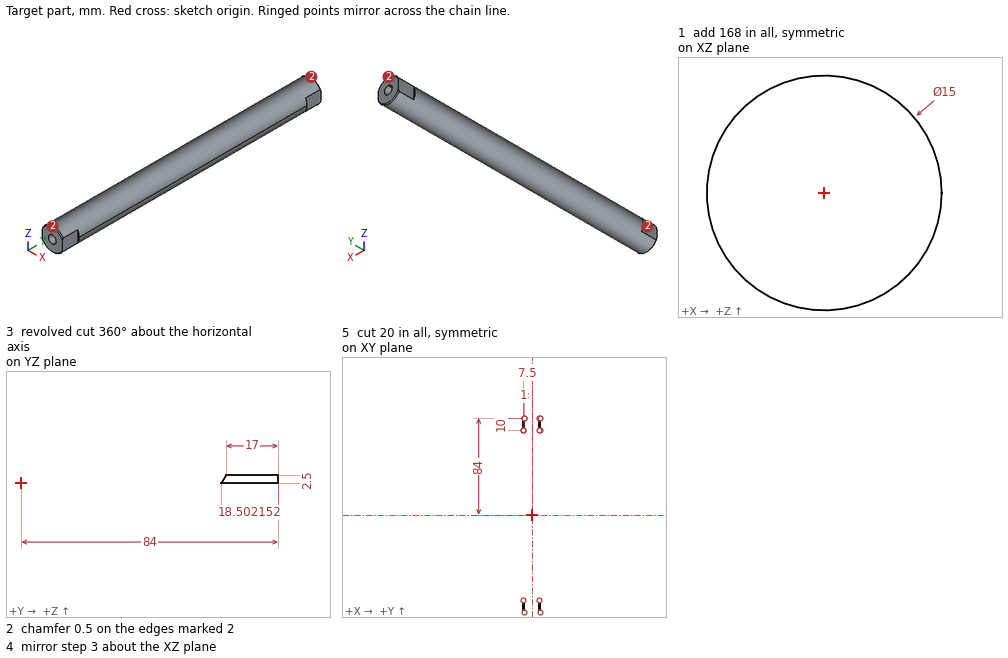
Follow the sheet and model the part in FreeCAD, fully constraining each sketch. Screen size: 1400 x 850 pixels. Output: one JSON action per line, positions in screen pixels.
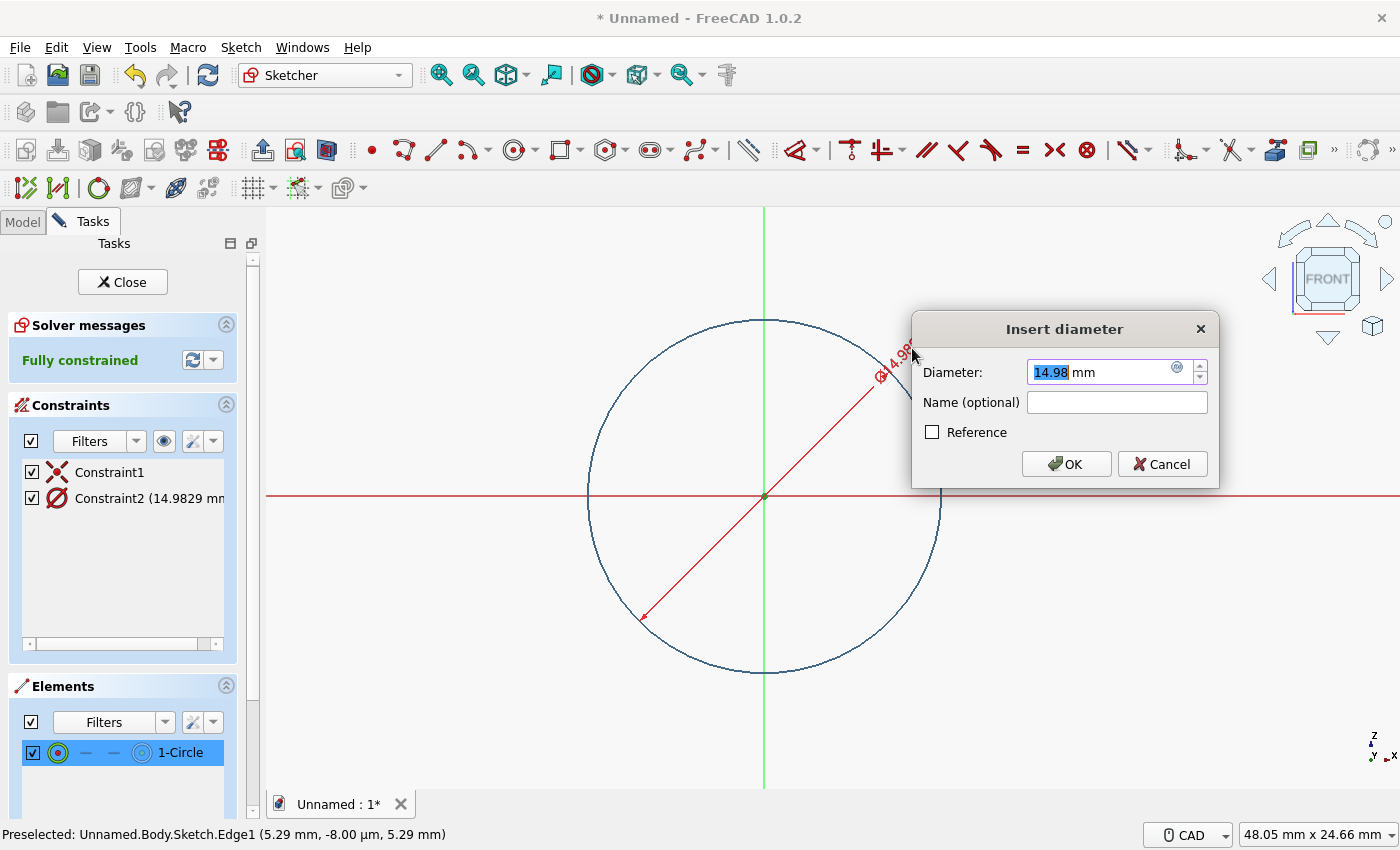
{"action": "type", "text": "15"}
{"action": "key", "text": "Return"}
{"action": "key", "text": "Escape"}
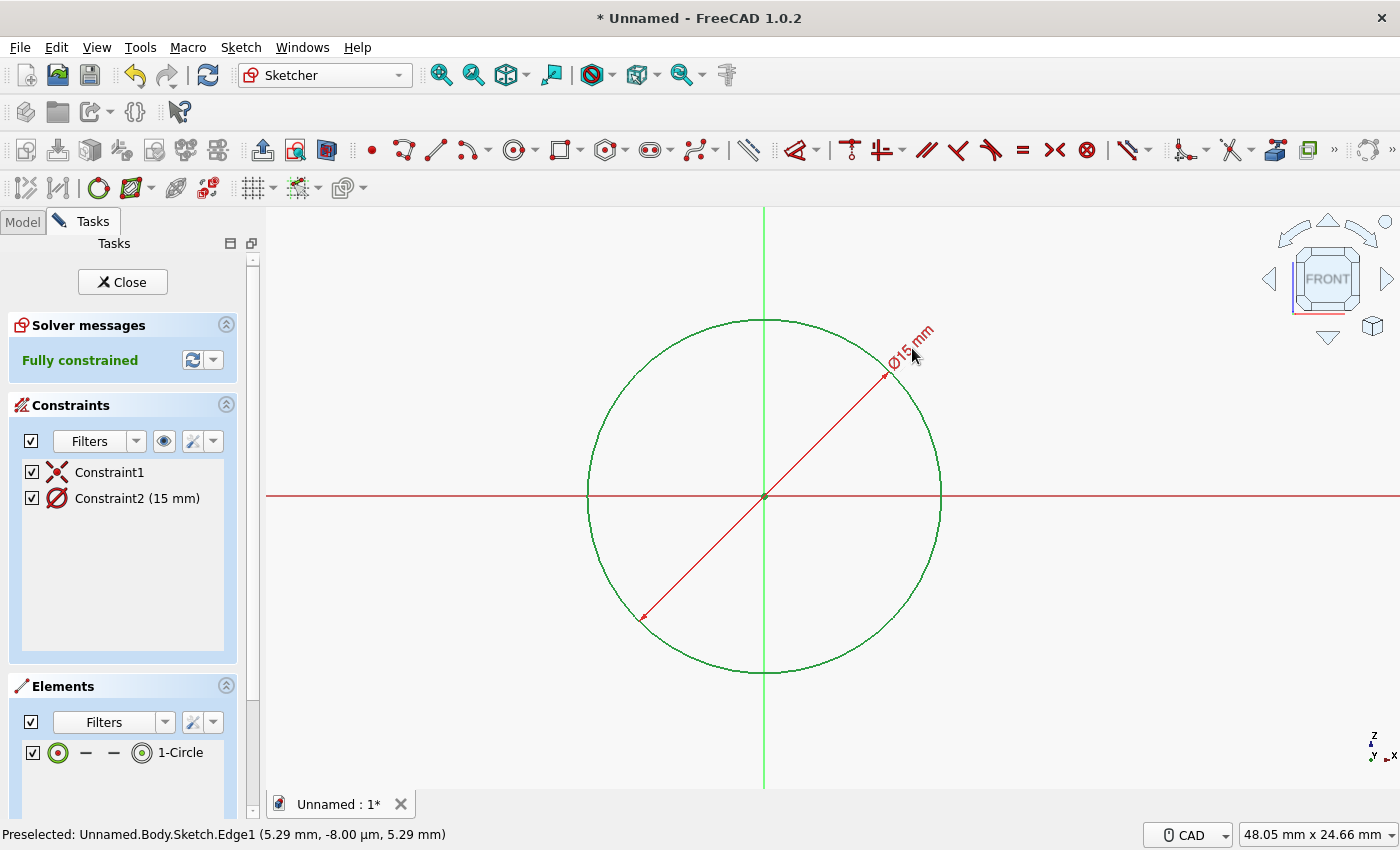
{"action": "left_click", "coordinate": [123, 282]}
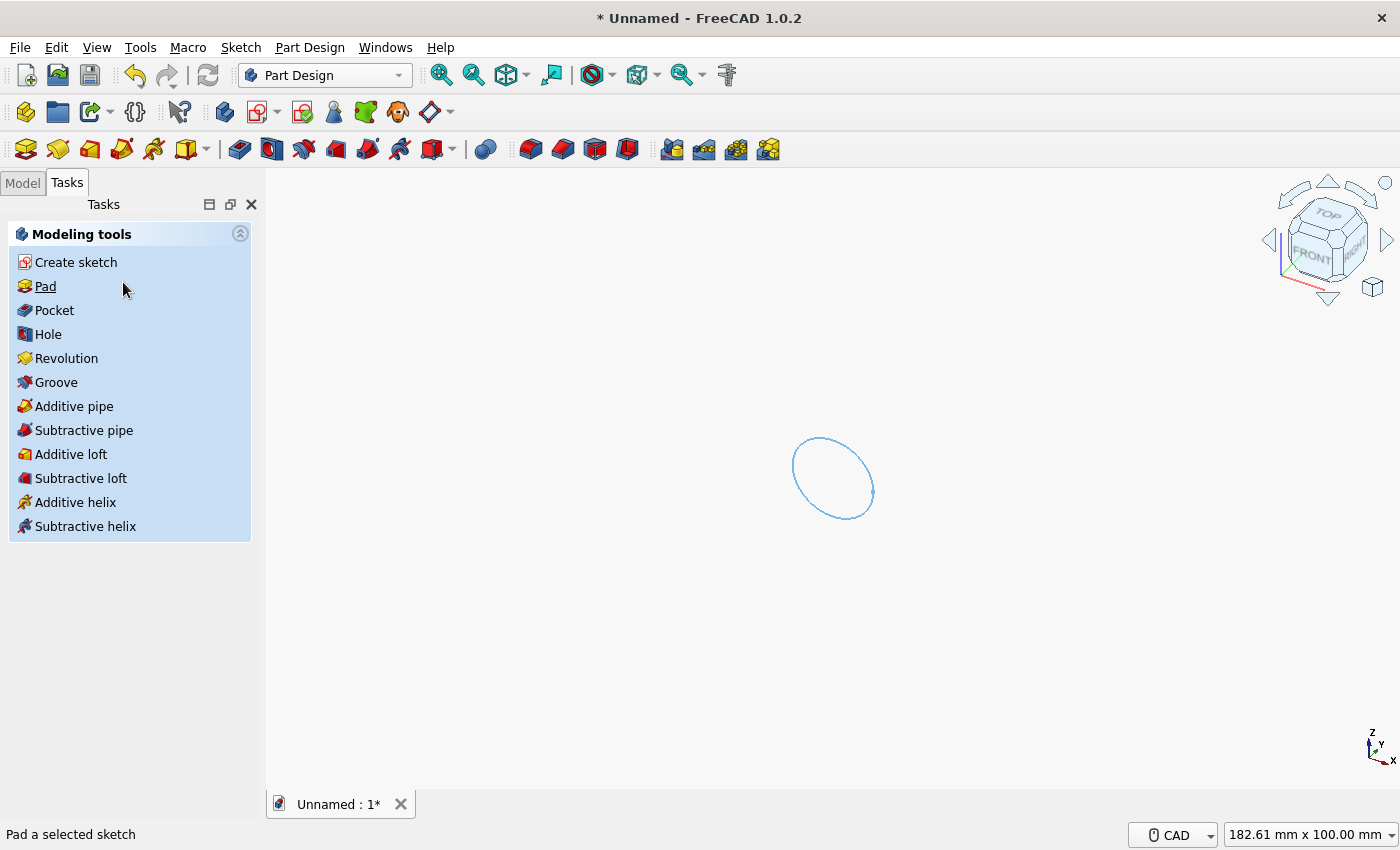
{"action": "left_click", "coordinate": [26, 150]}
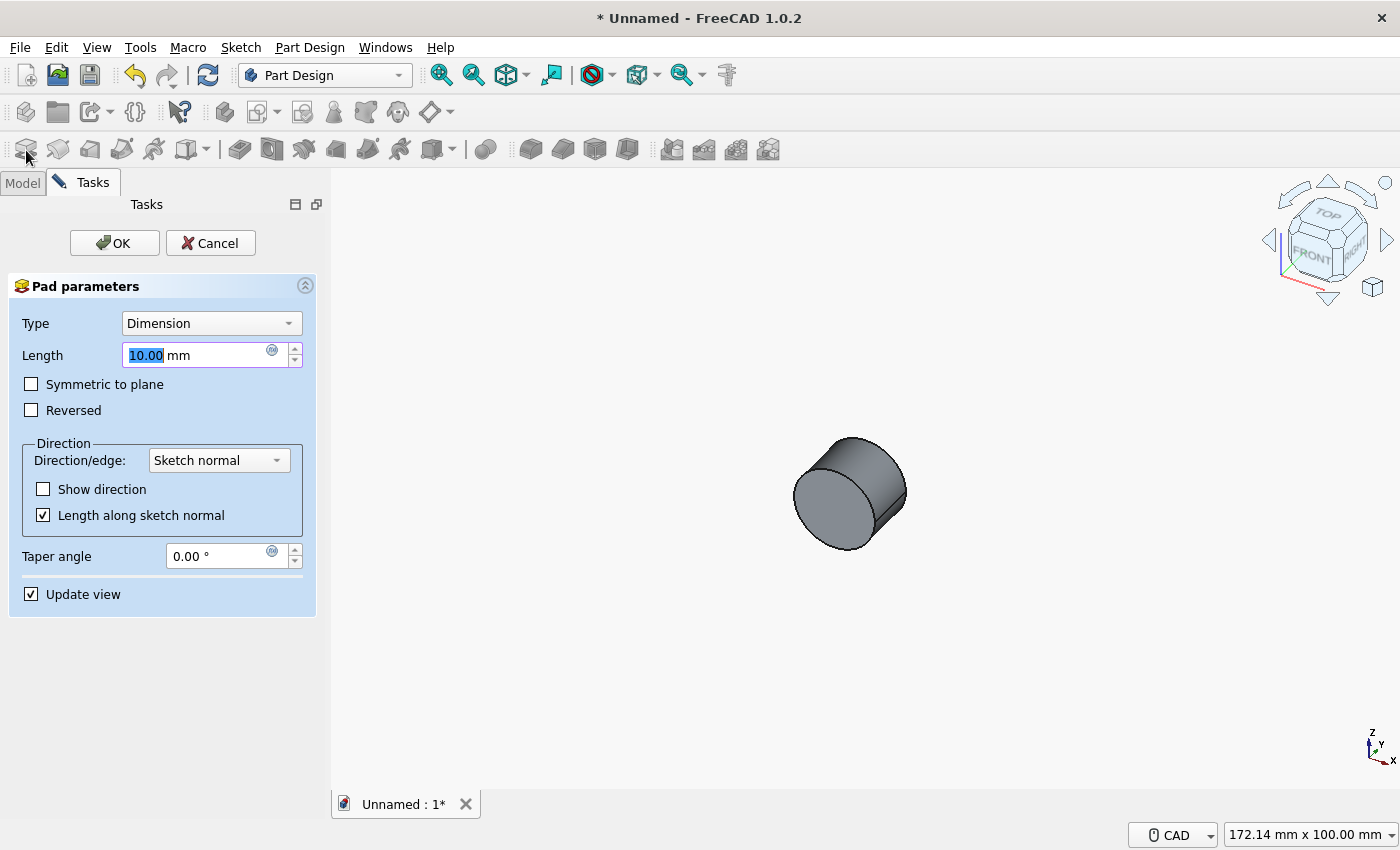
{"action": "type", "text": "168"}
{"action": "key", "text": "Tab"}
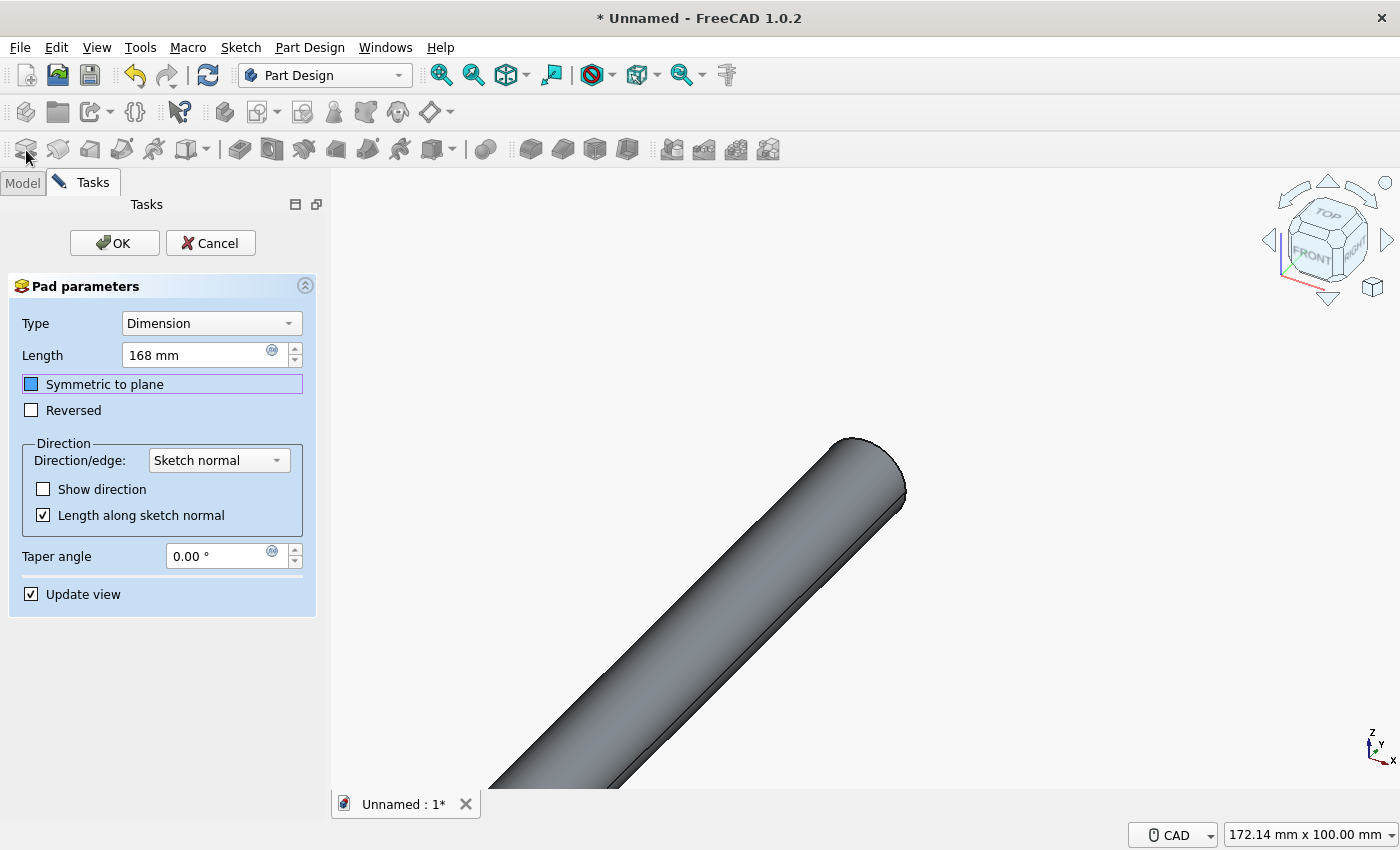
{"action": "left_click", "coordinate": [30, 384]}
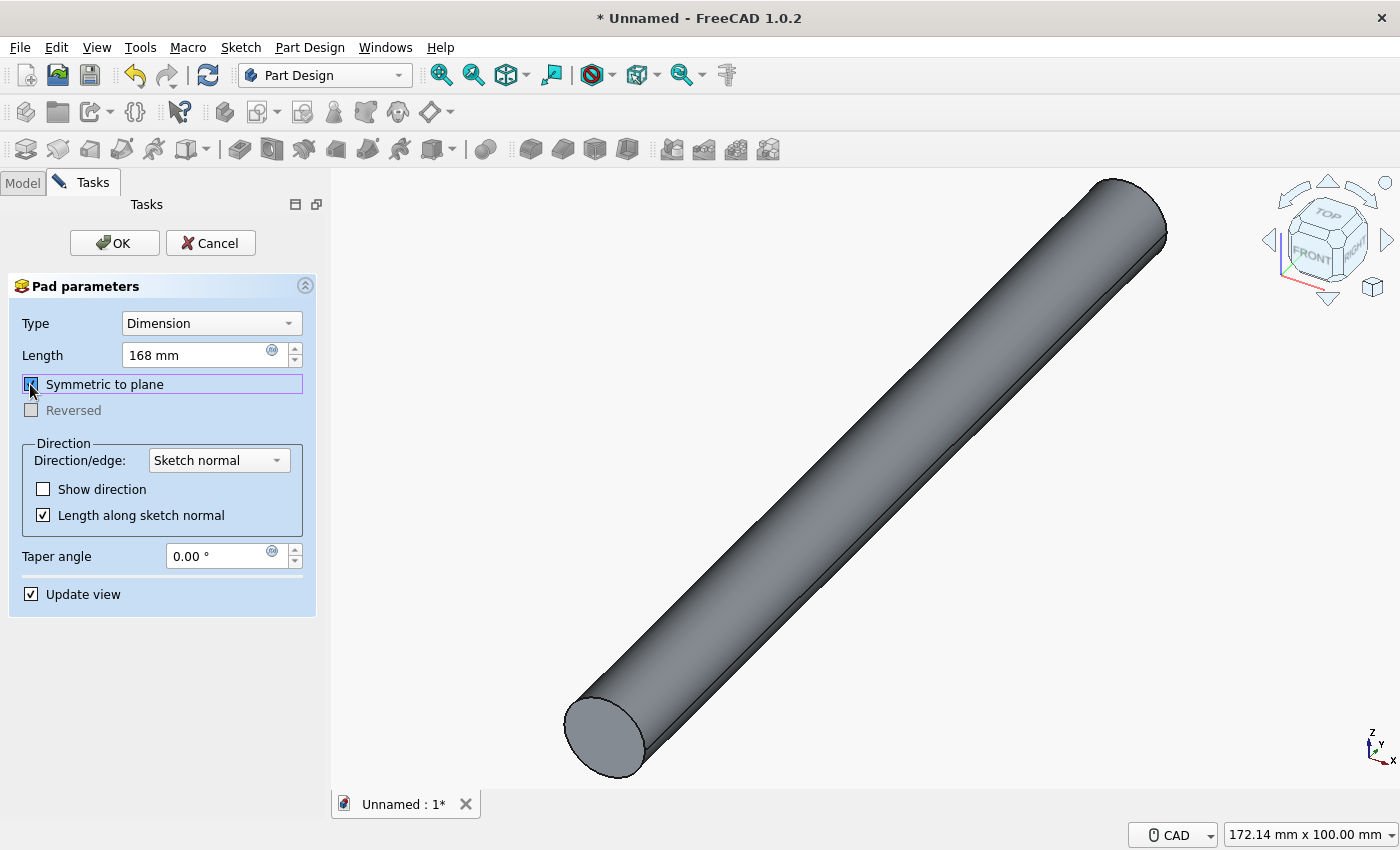
{"action": "left_click", "coordinate": [115, 243]}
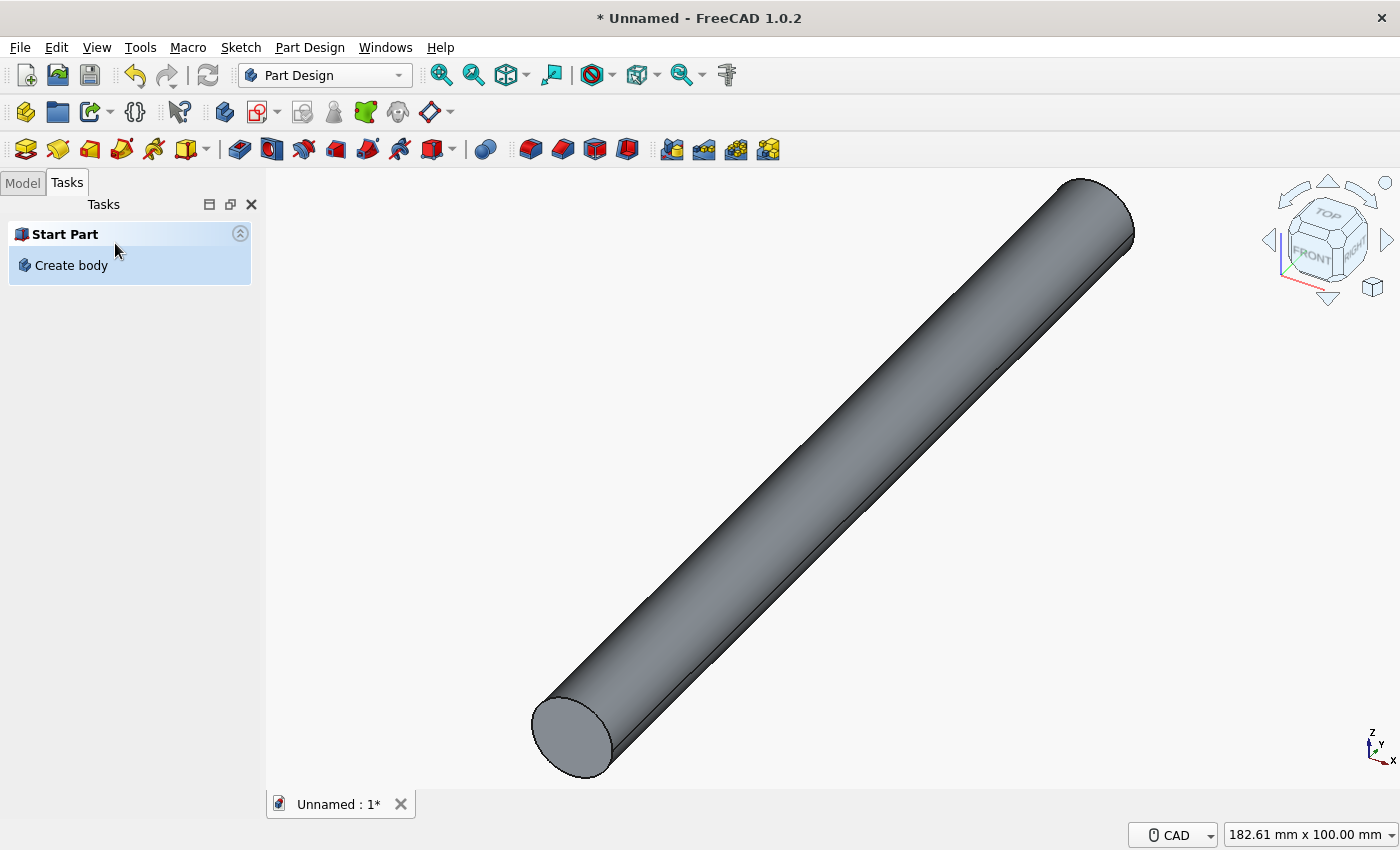
{"action": "left_click", "coordinate": [442, 76]}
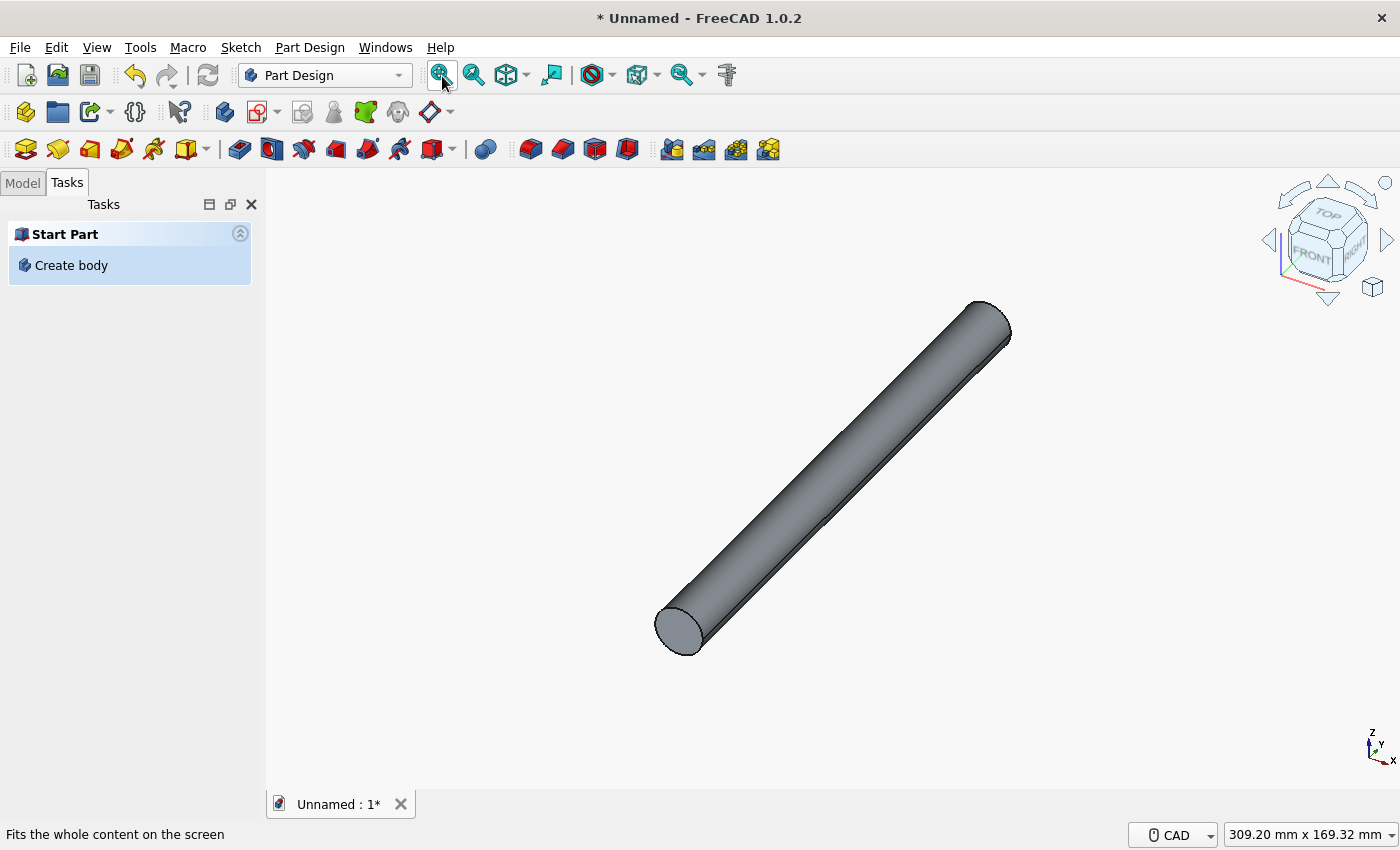
{"action": "left_click", "coordinate": [660, 611]}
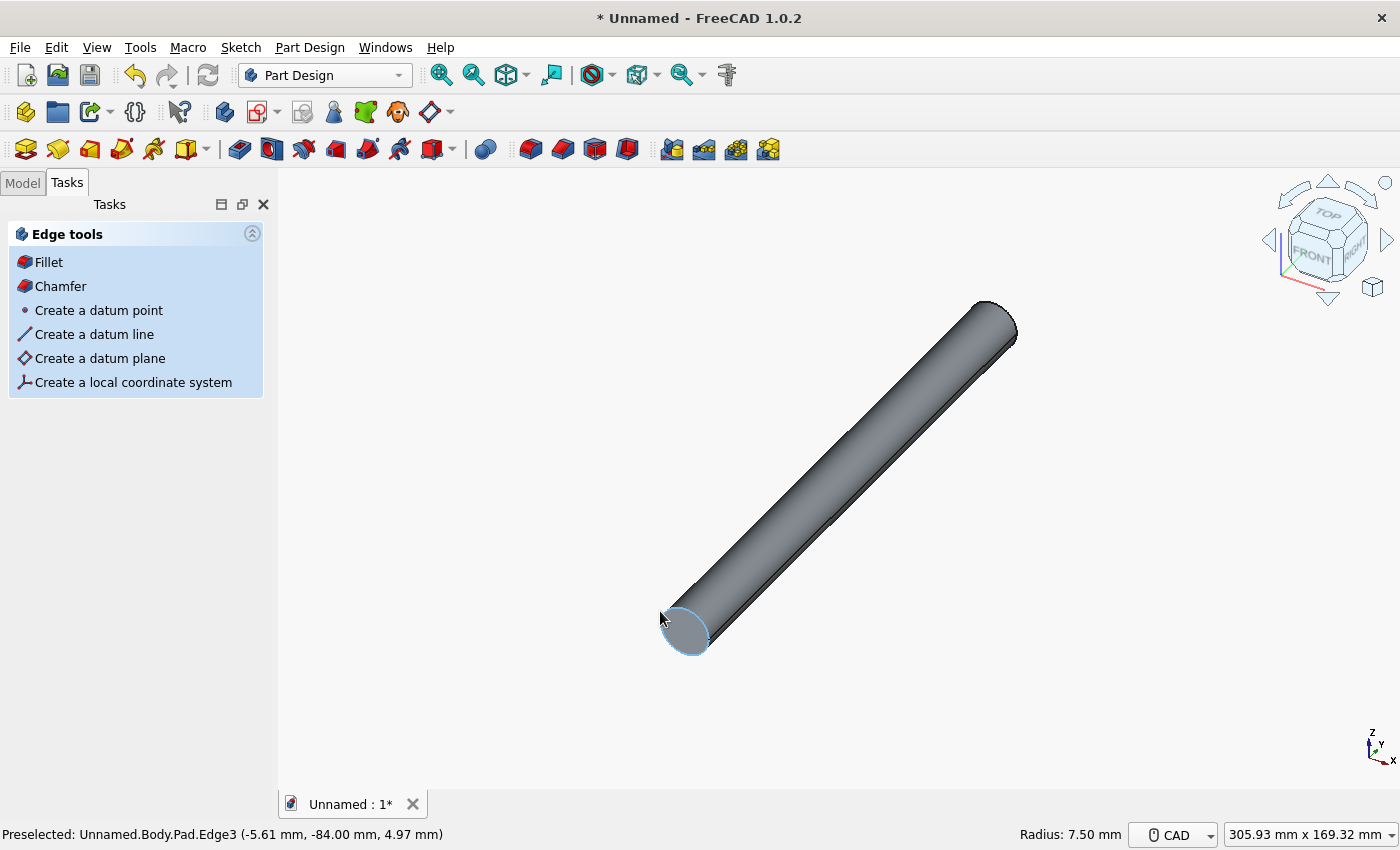
{"action": "key", "text": "0"}